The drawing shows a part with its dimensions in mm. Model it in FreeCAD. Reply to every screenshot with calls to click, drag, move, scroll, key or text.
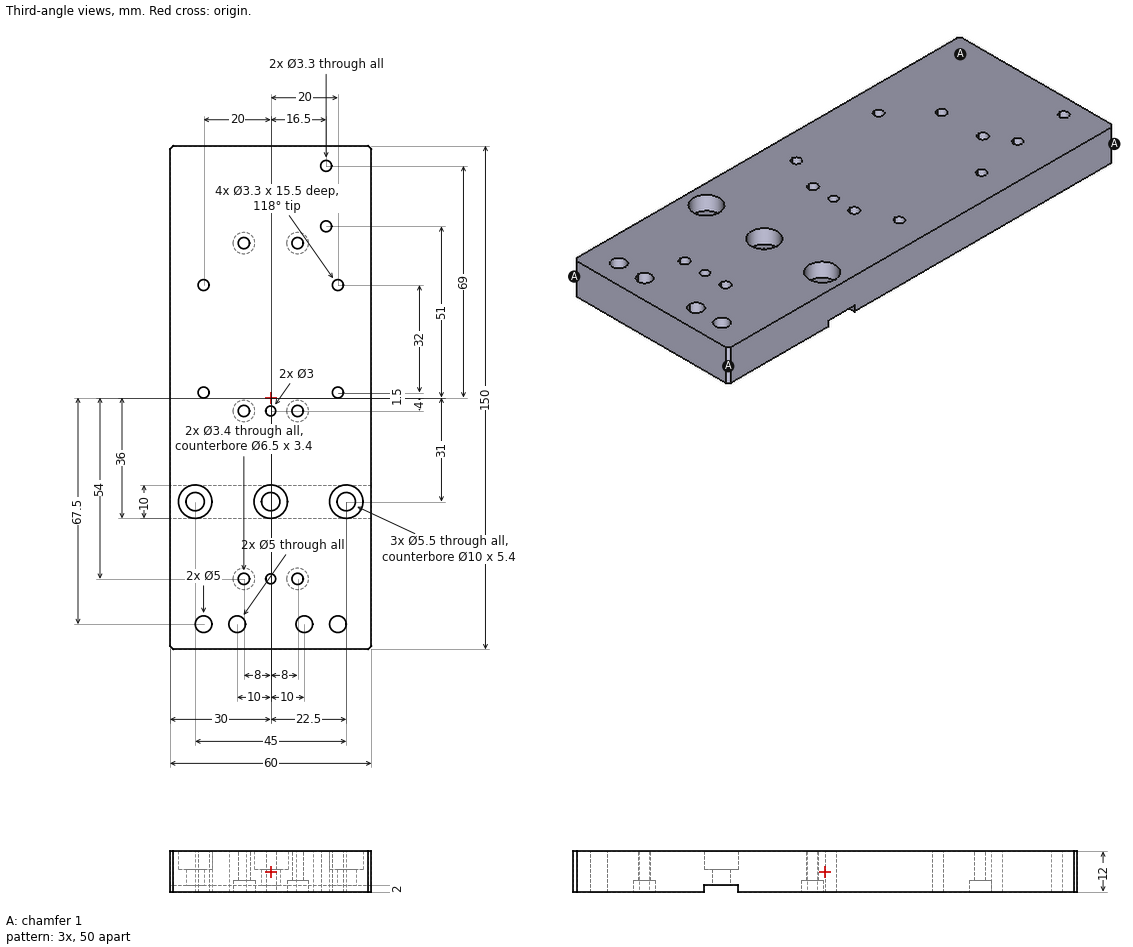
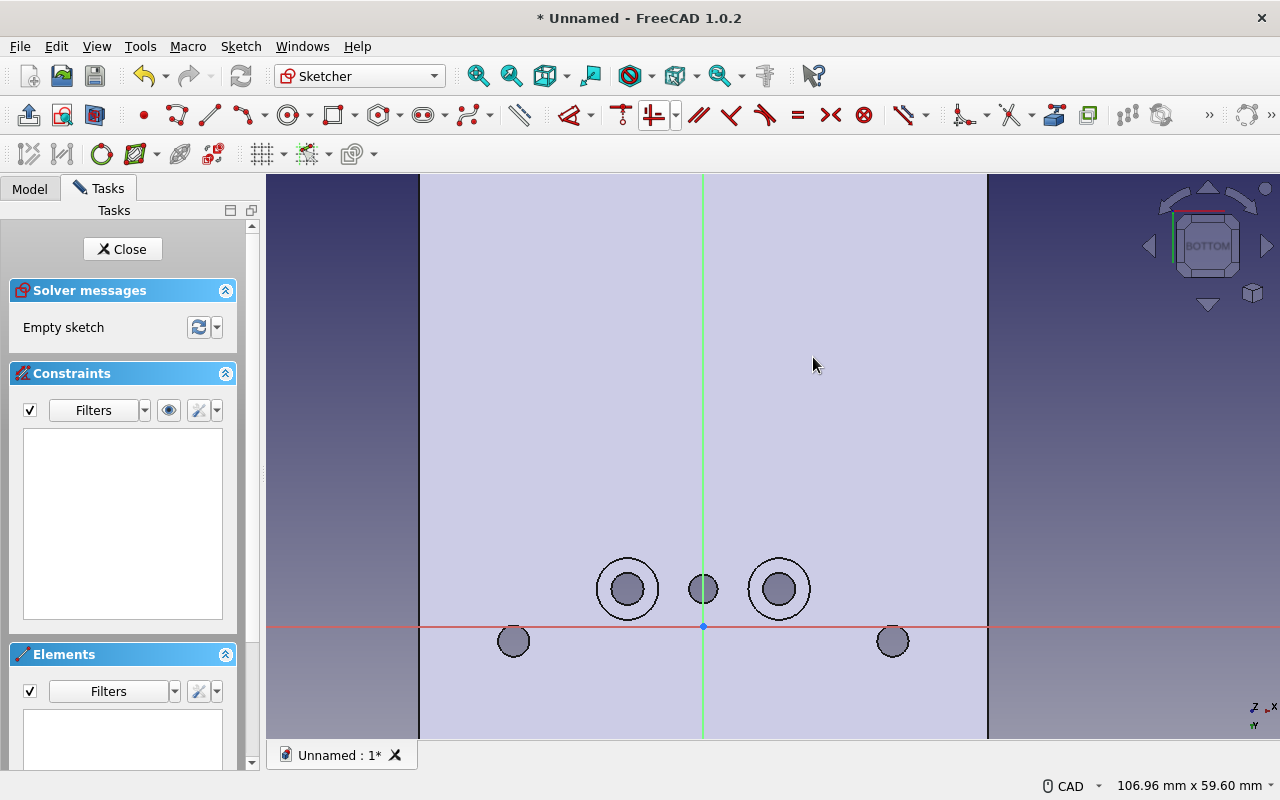
click(332, 116)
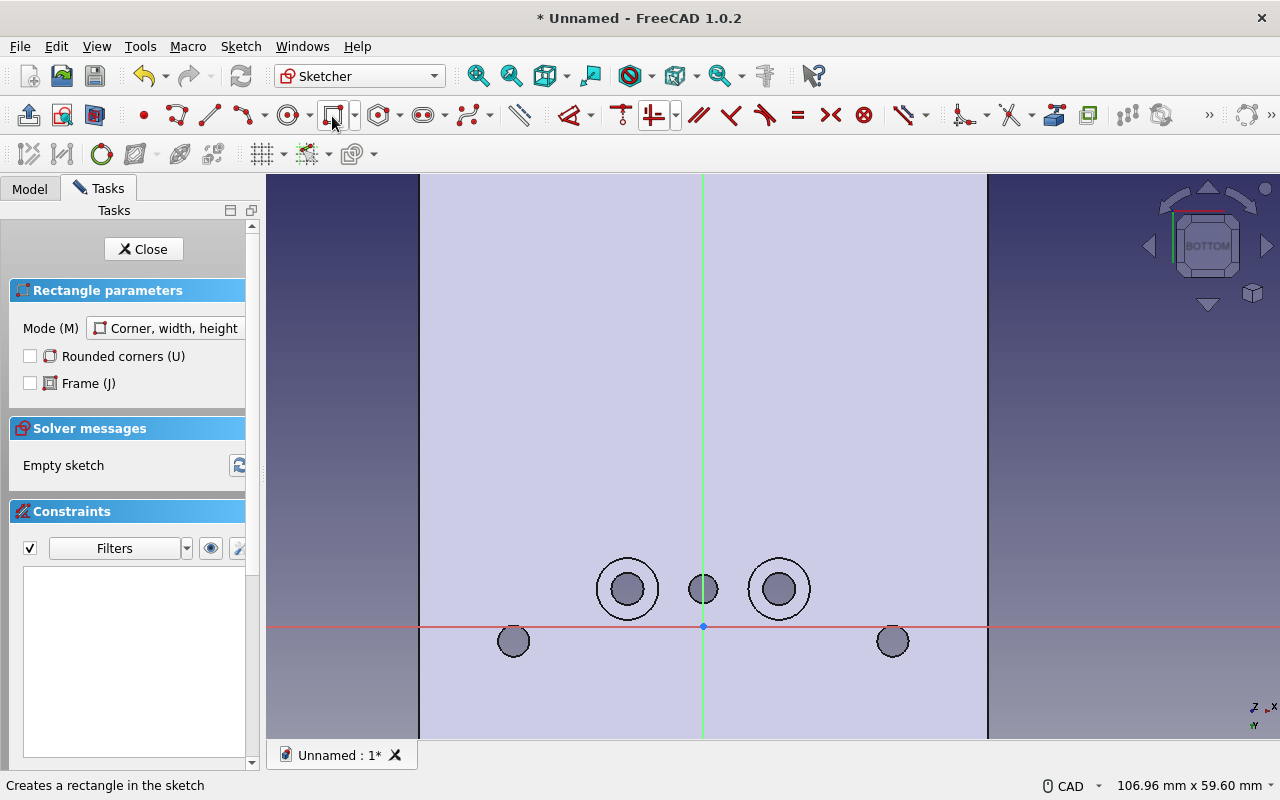
click(419, 286)
click(988, 380)
key(Escape)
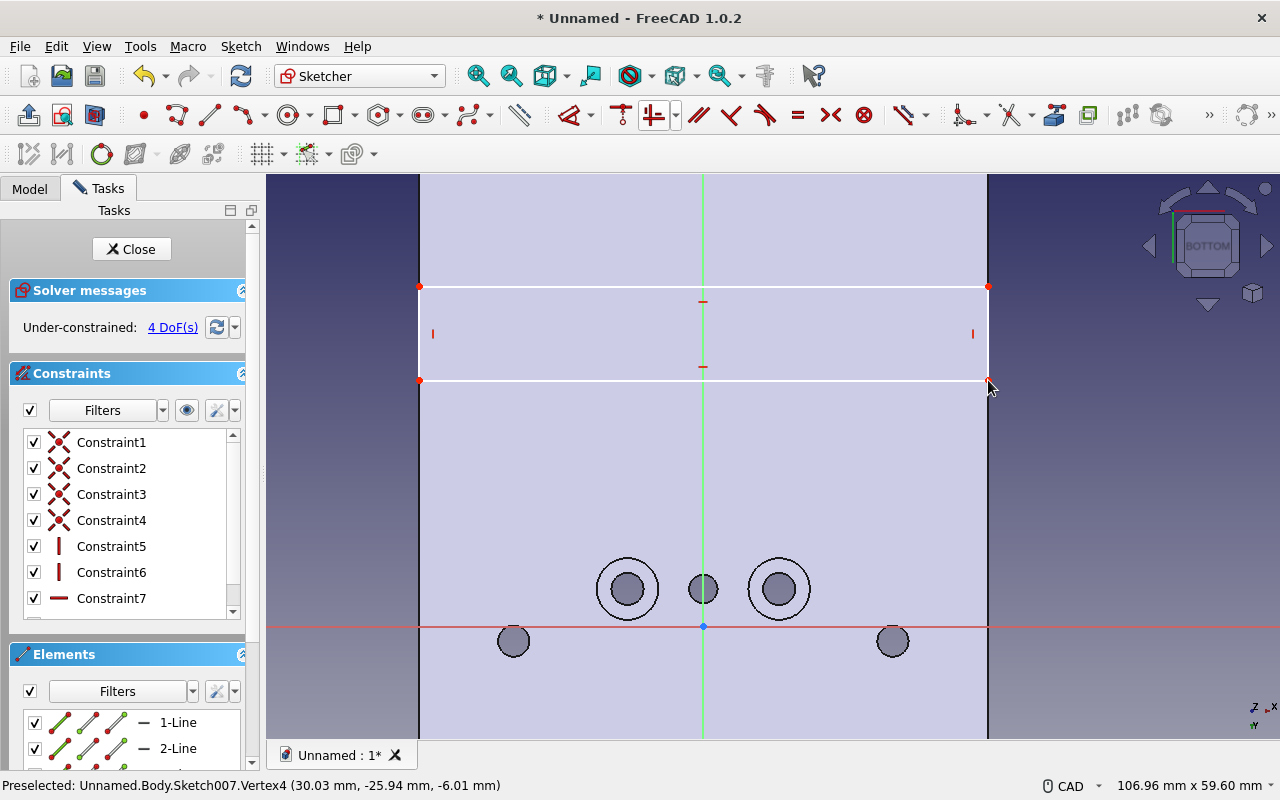
click(568, 116)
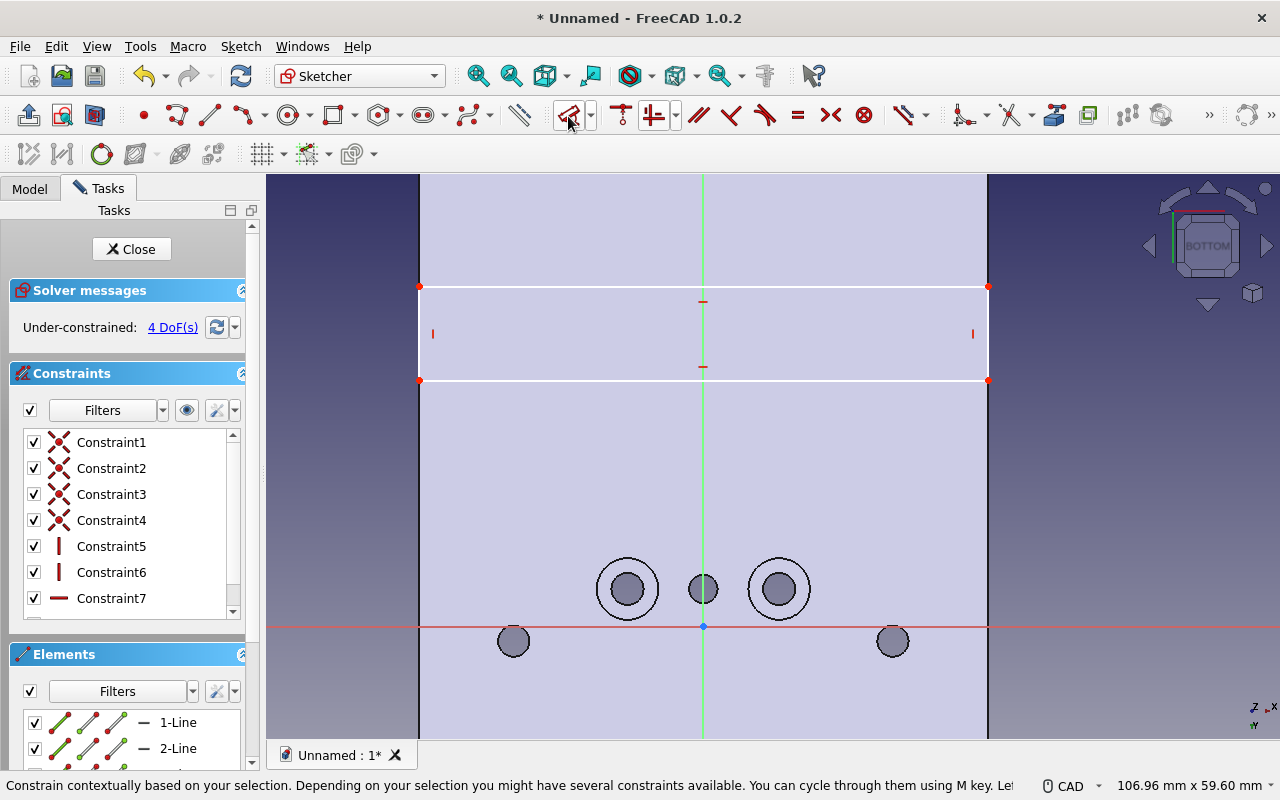
click(419, 315)
click(385, 334)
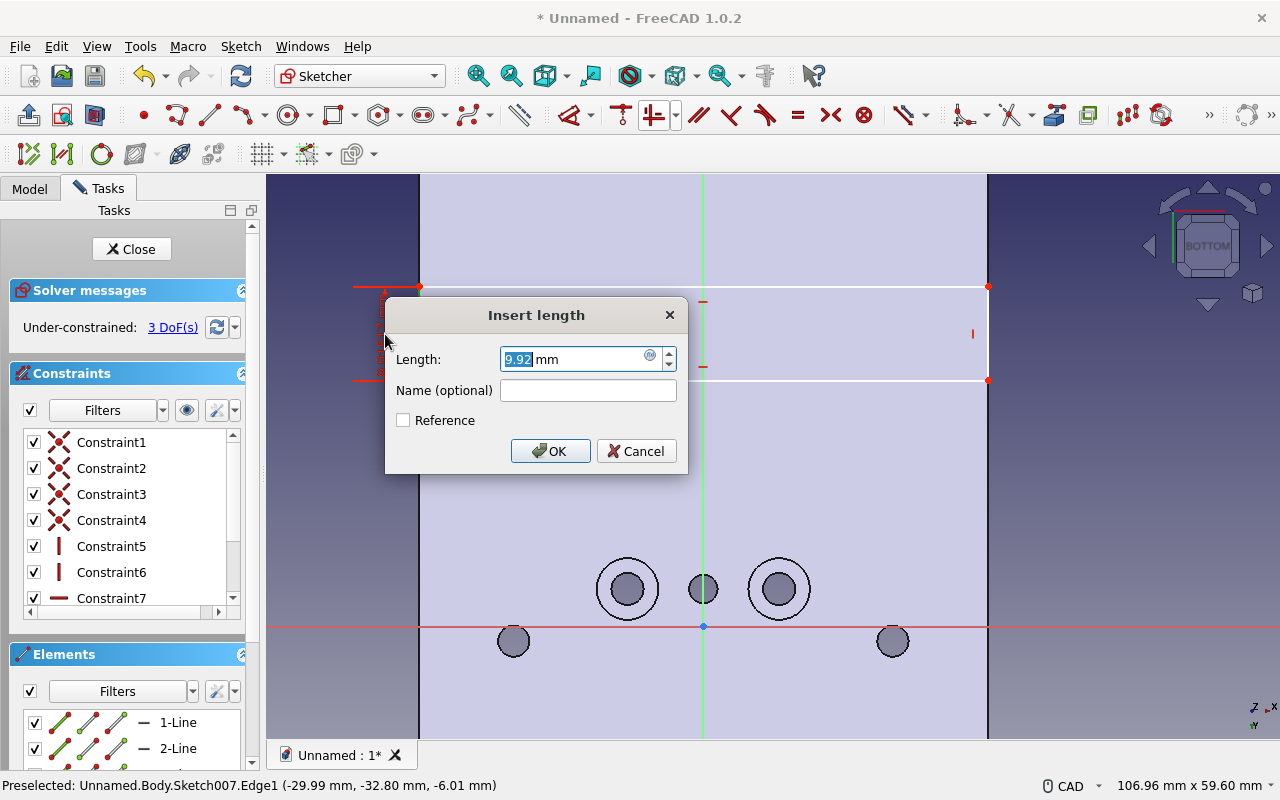
text(10)
key(Return)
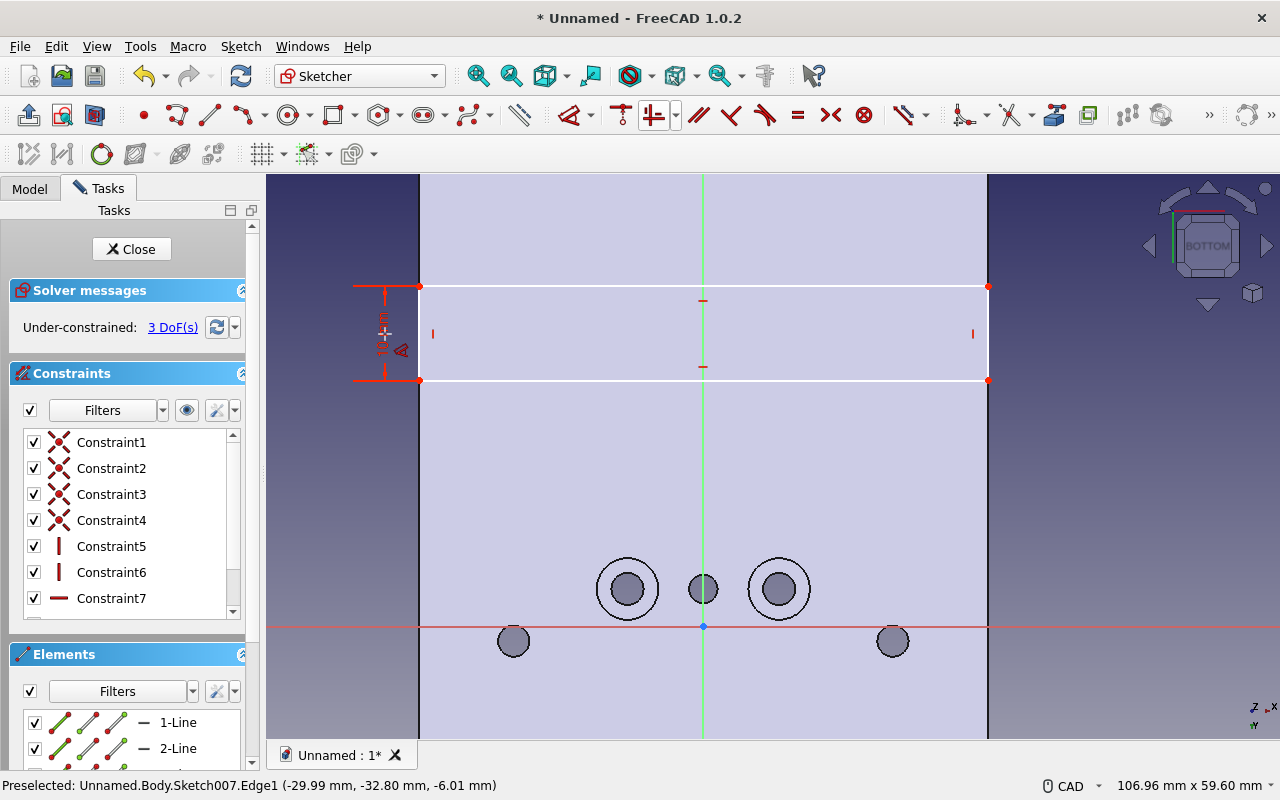
click(590, 381)
click(573, 347)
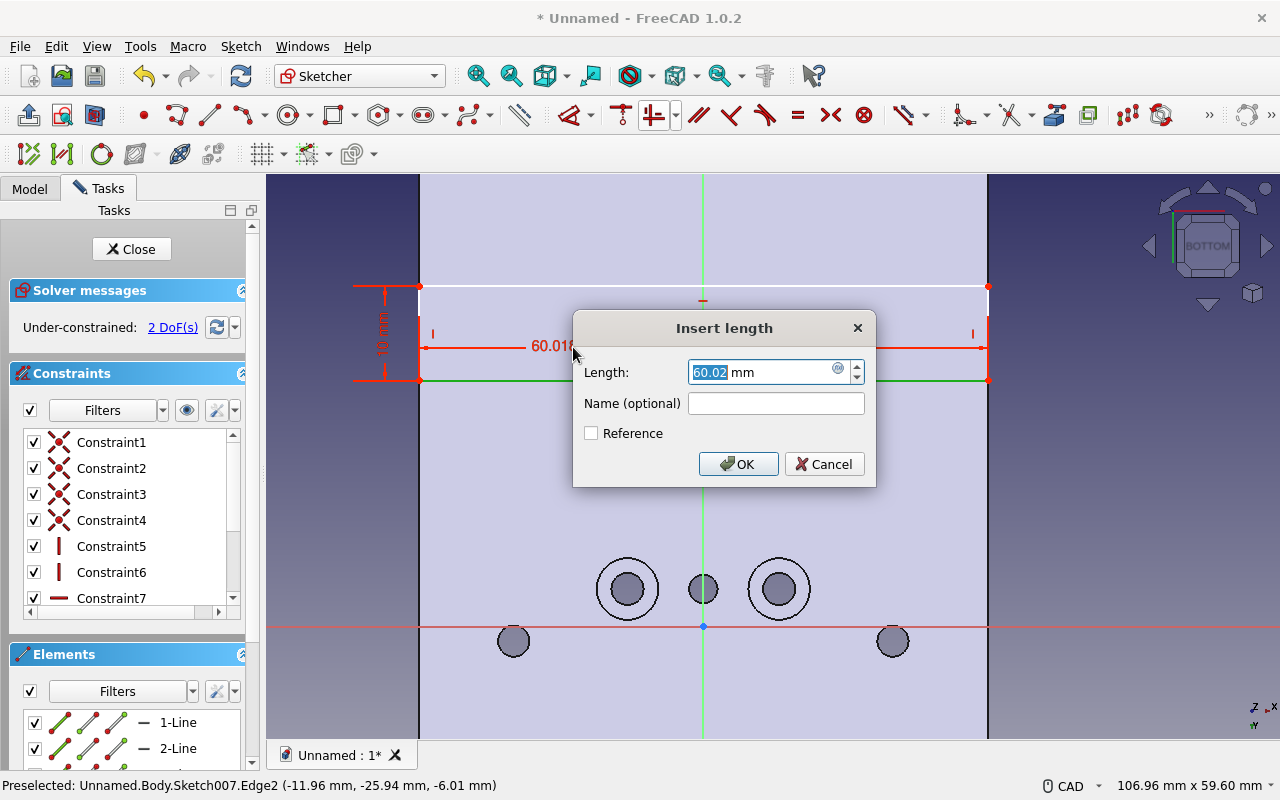
text(60)
key(Return)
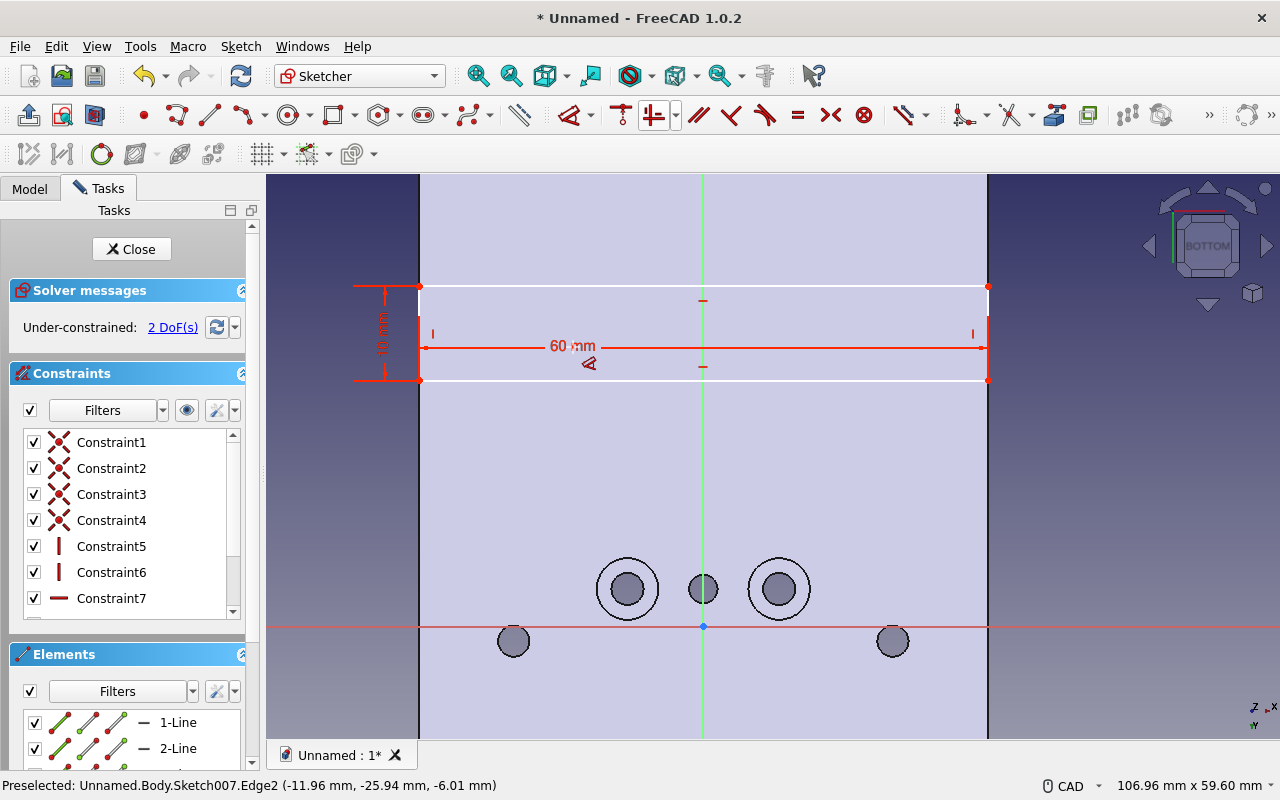
click(419, 286)
click(561, 661)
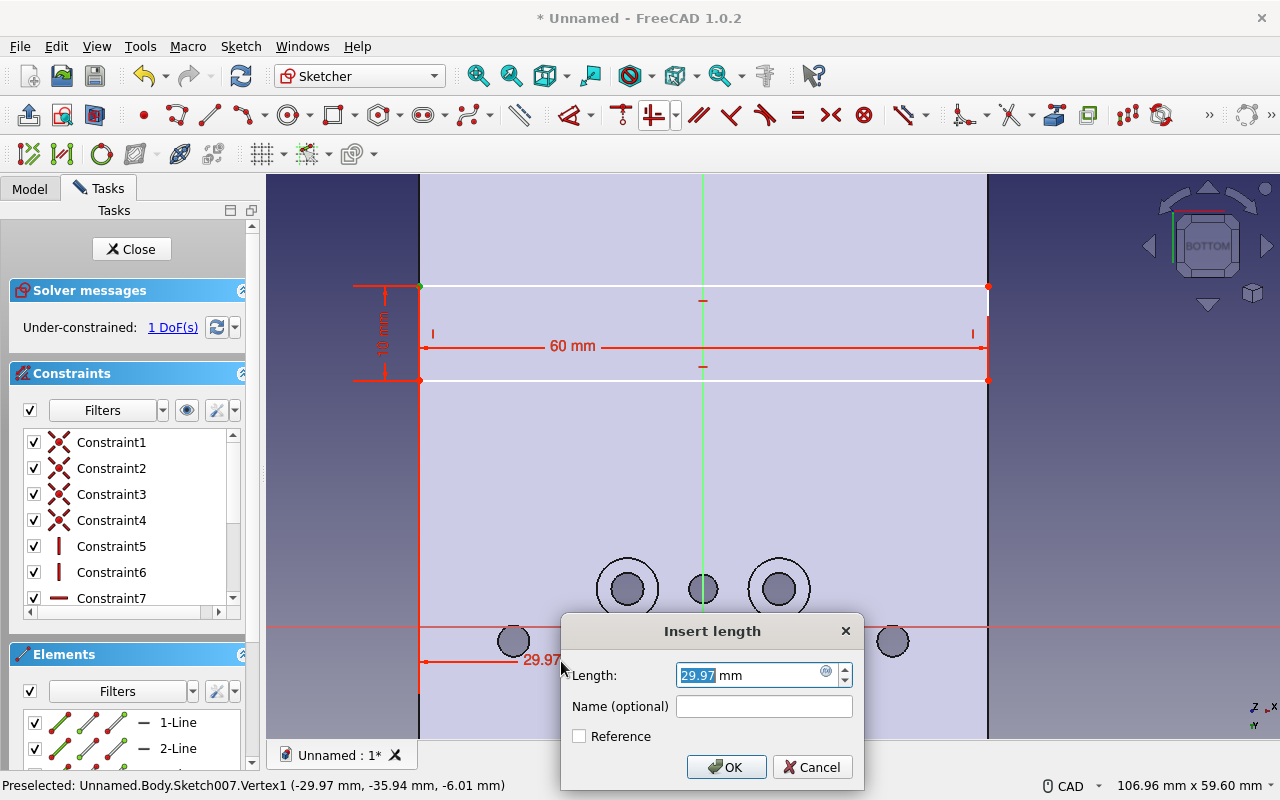
text(30)
key(Return)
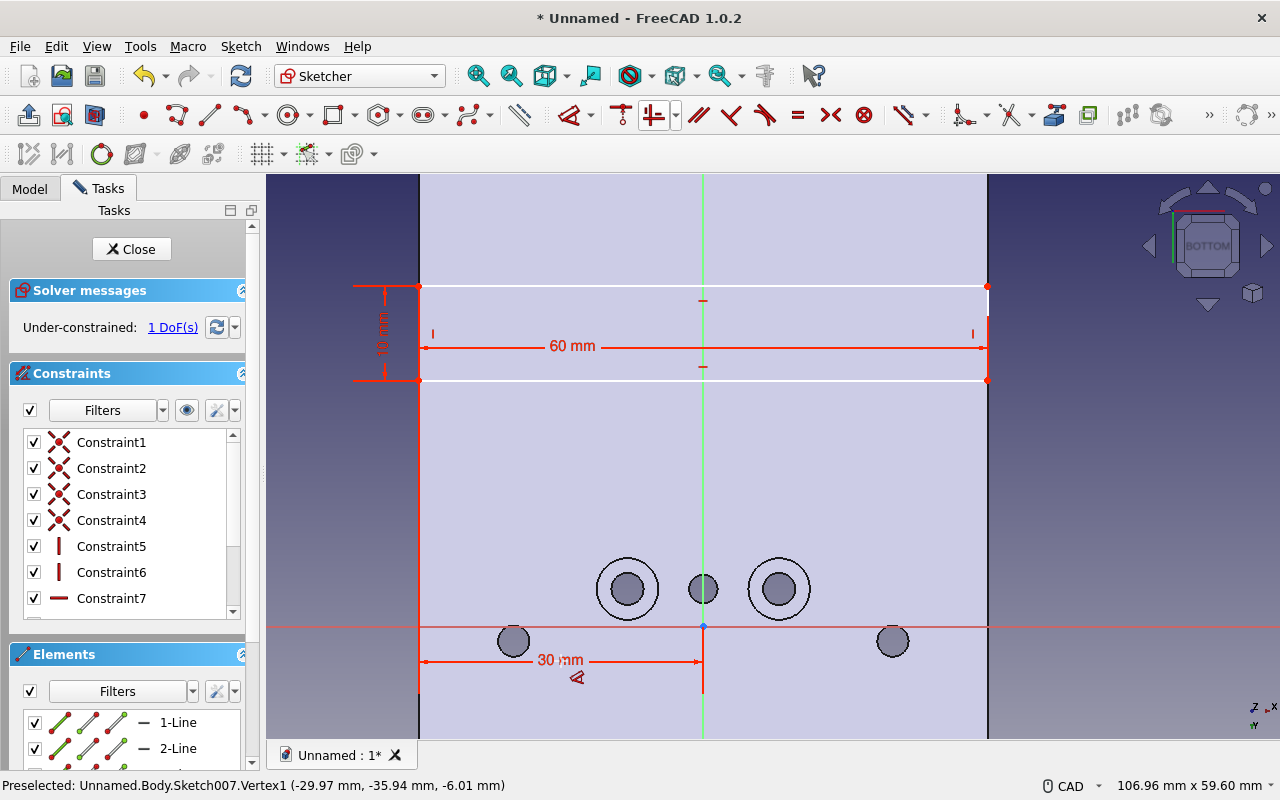
click(419, 286)
click(385, 457)